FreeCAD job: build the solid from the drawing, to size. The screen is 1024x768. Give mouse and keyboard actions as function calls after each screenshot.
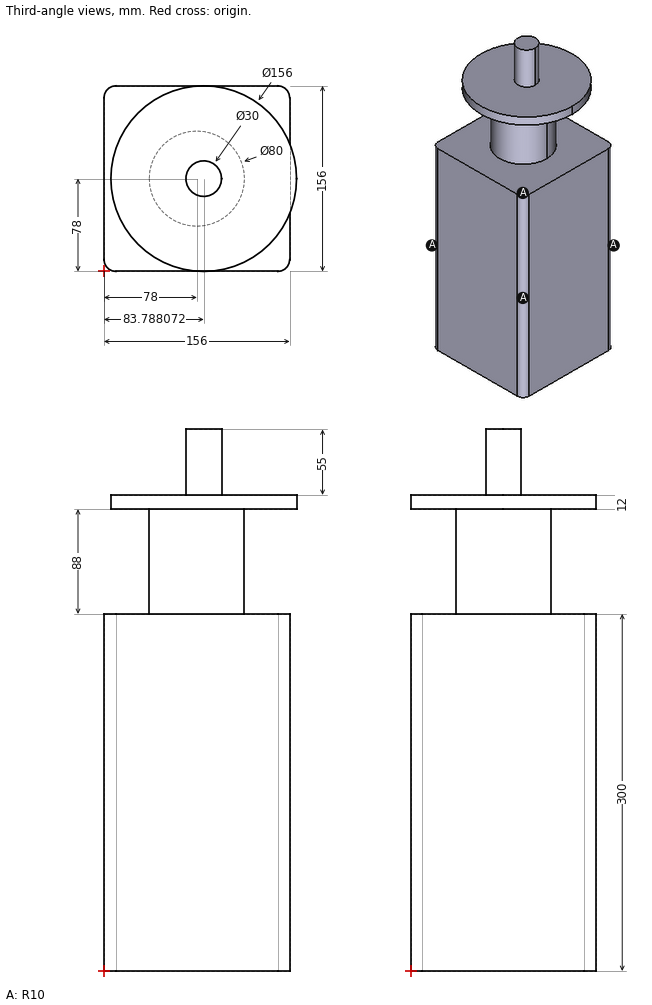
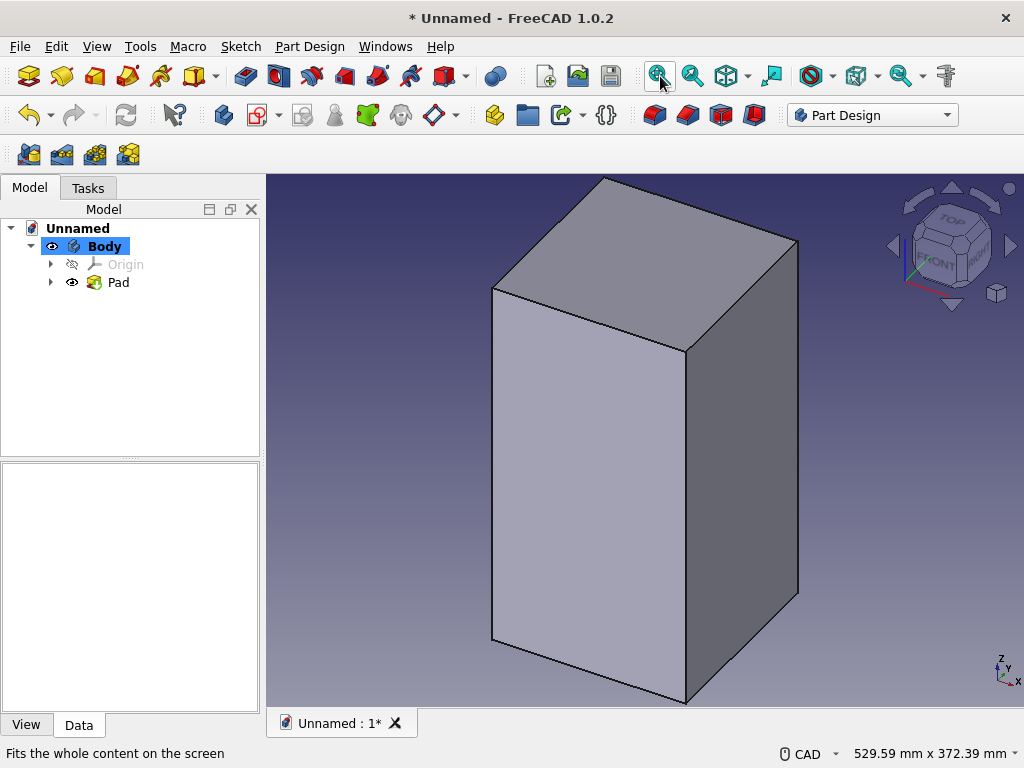
click(645, 264)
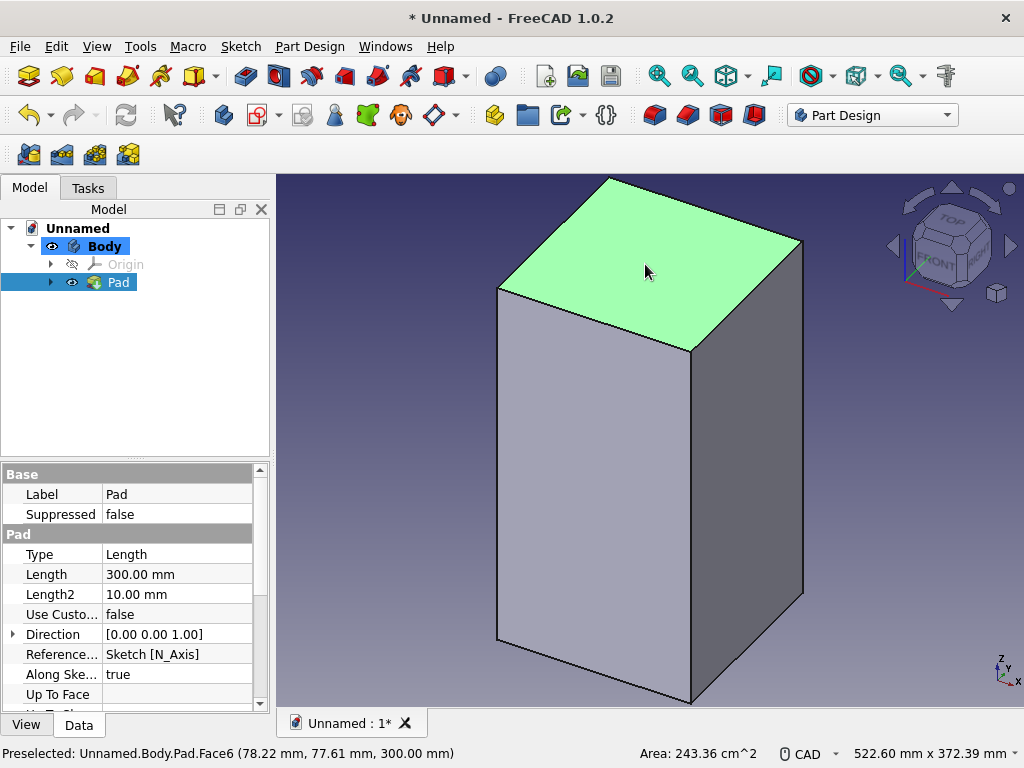
click(256, 116)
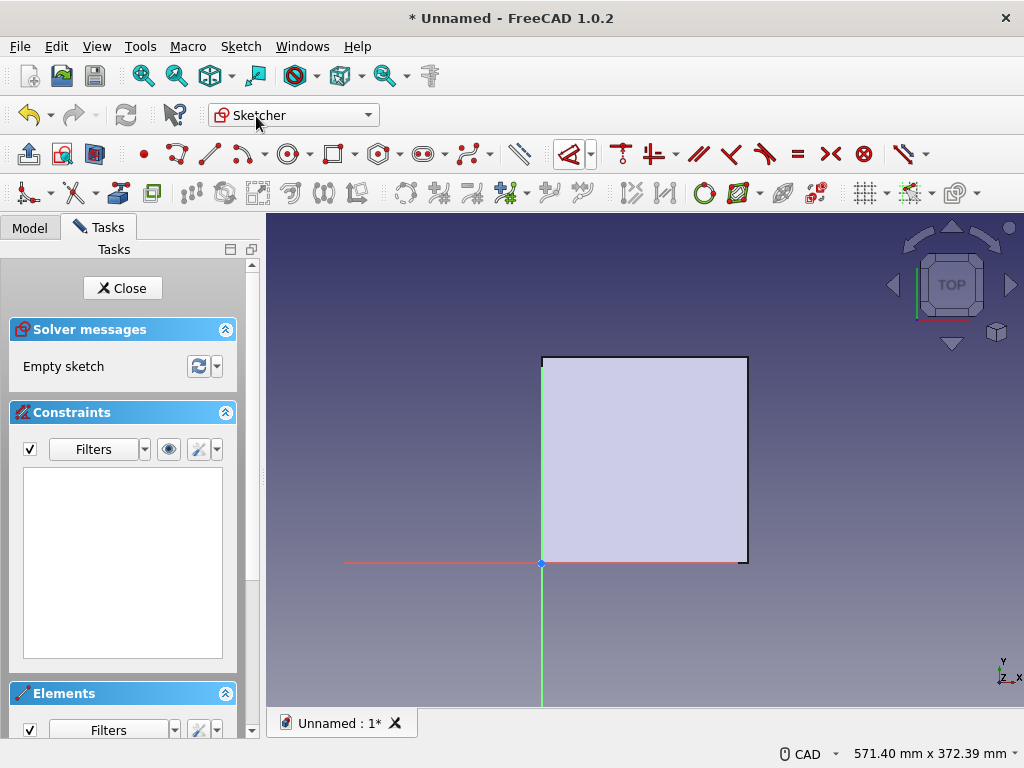
scroll(672, 516, up, 3)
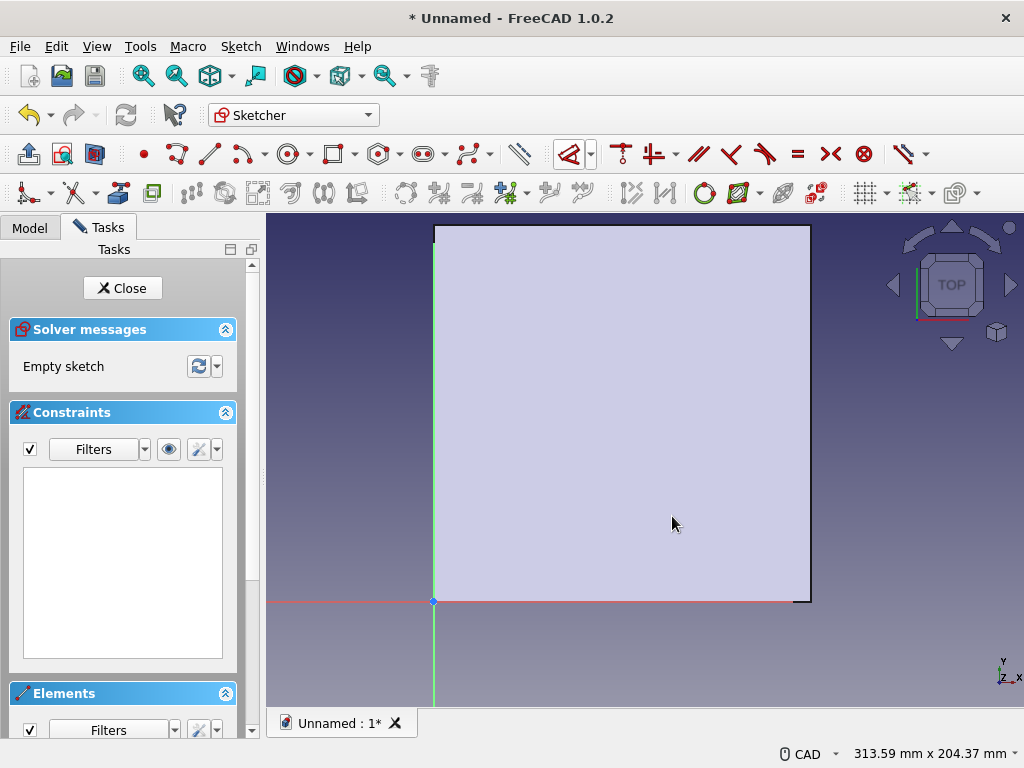
click(288, 154)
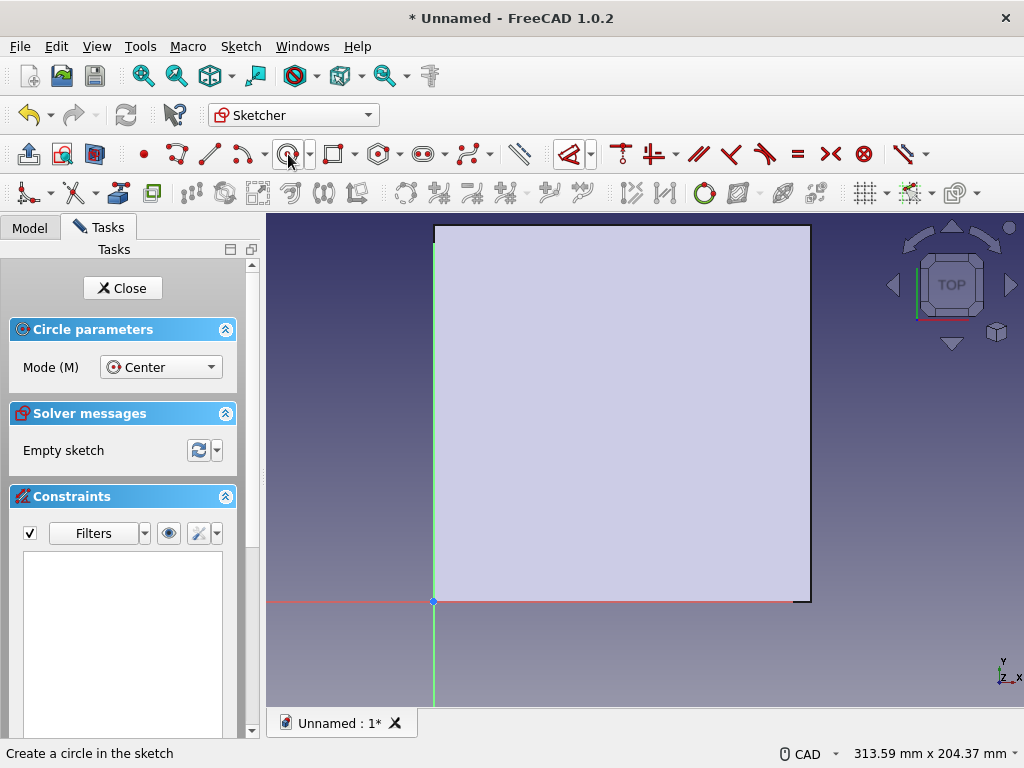
click(622, 413)
move(691, 345)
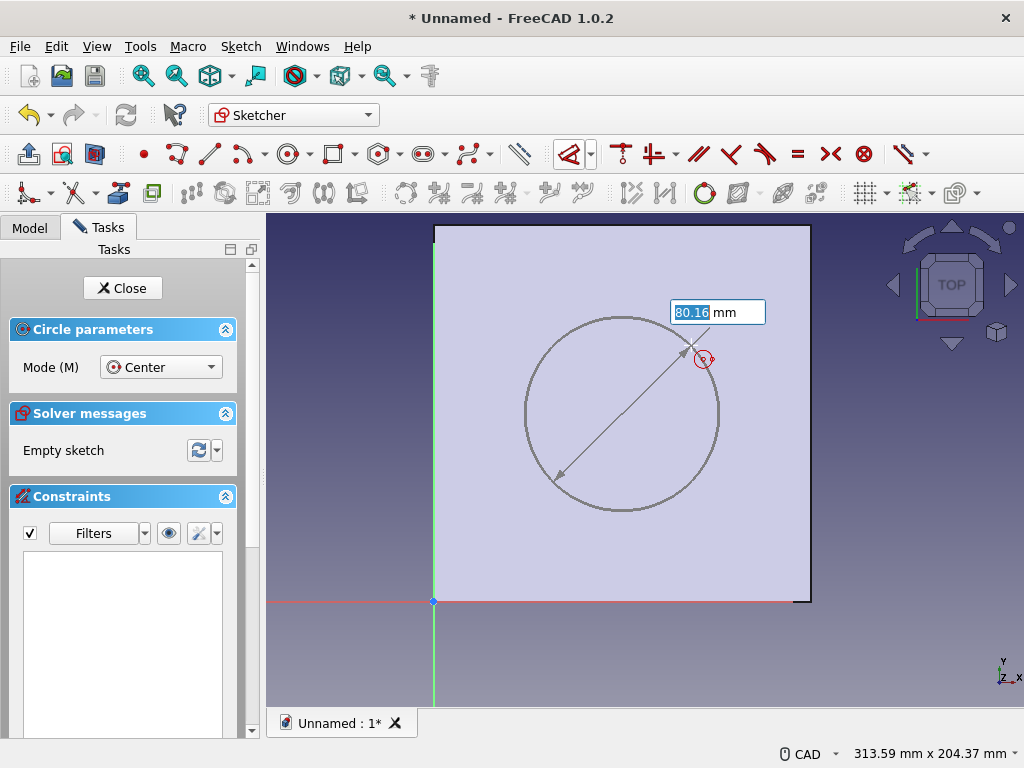
text(80)
key(Return)
key(Escape)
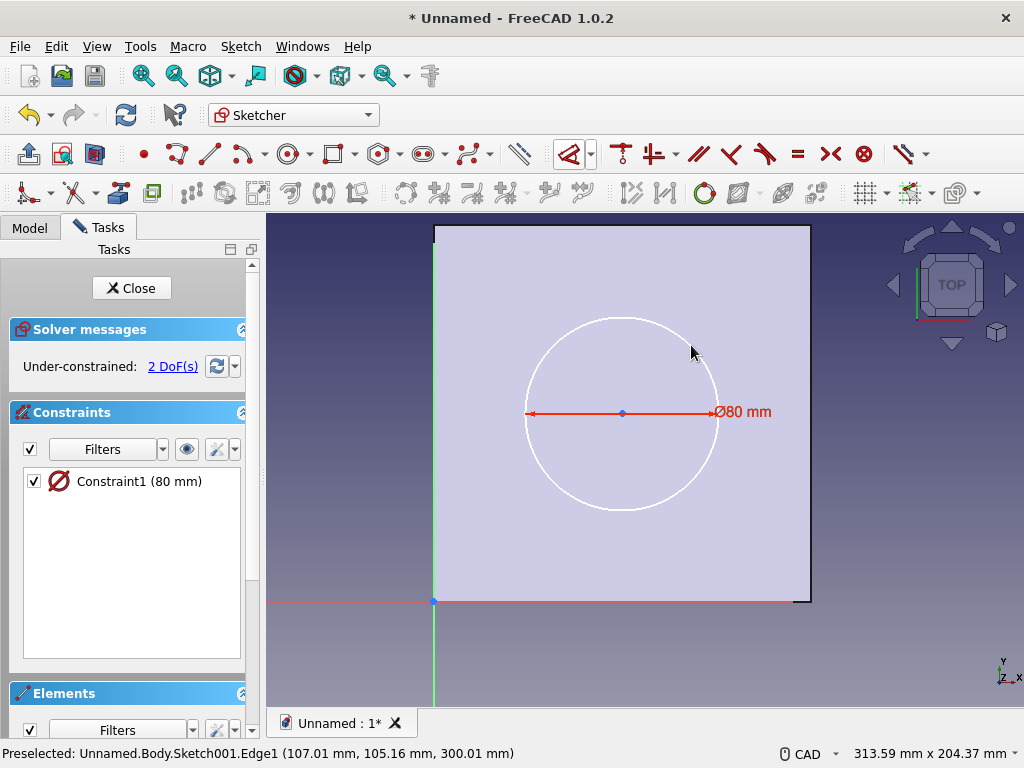
click(568, 154)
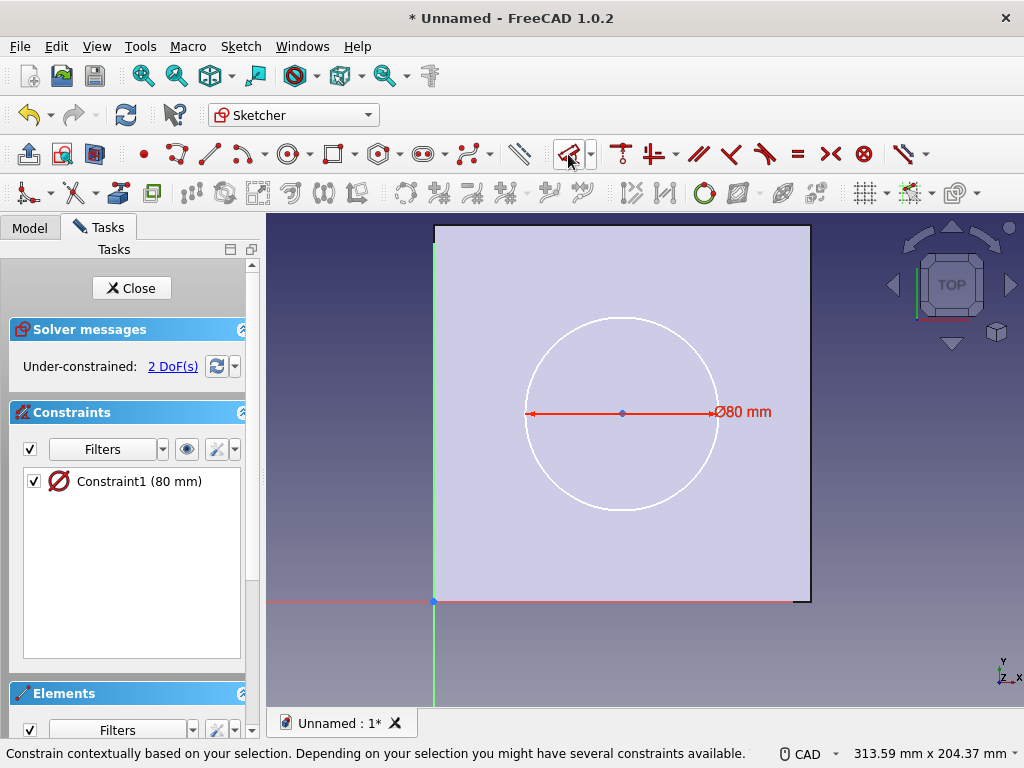
click(622, 414)
click(528, 636)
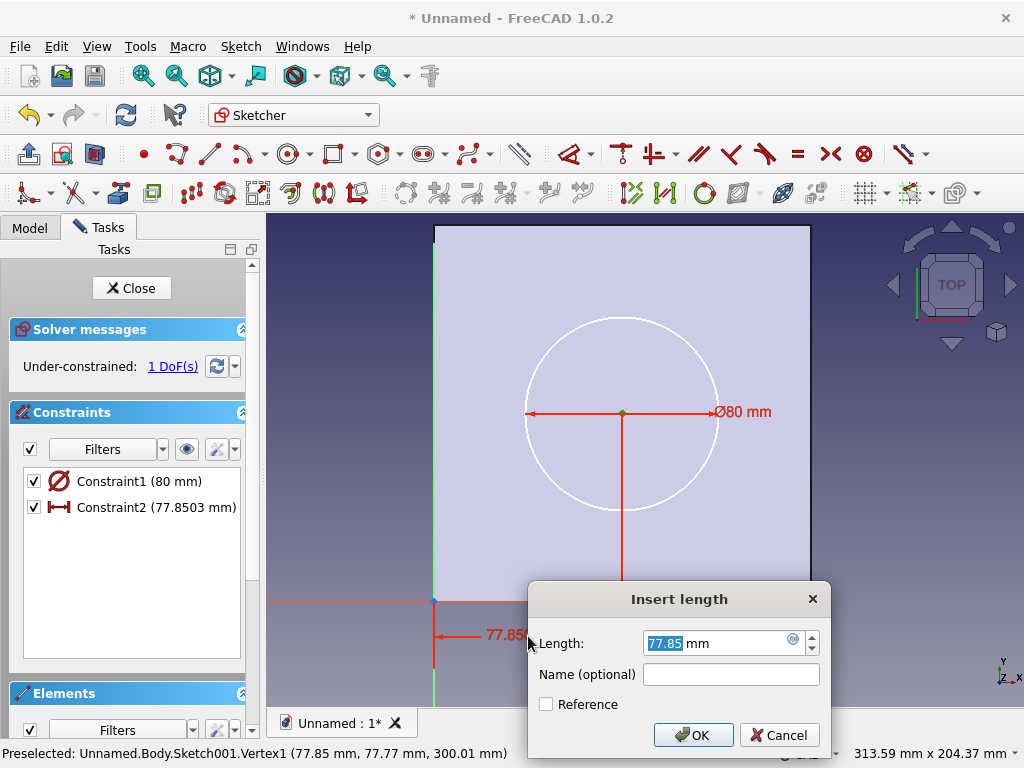
text(78)
key(Return)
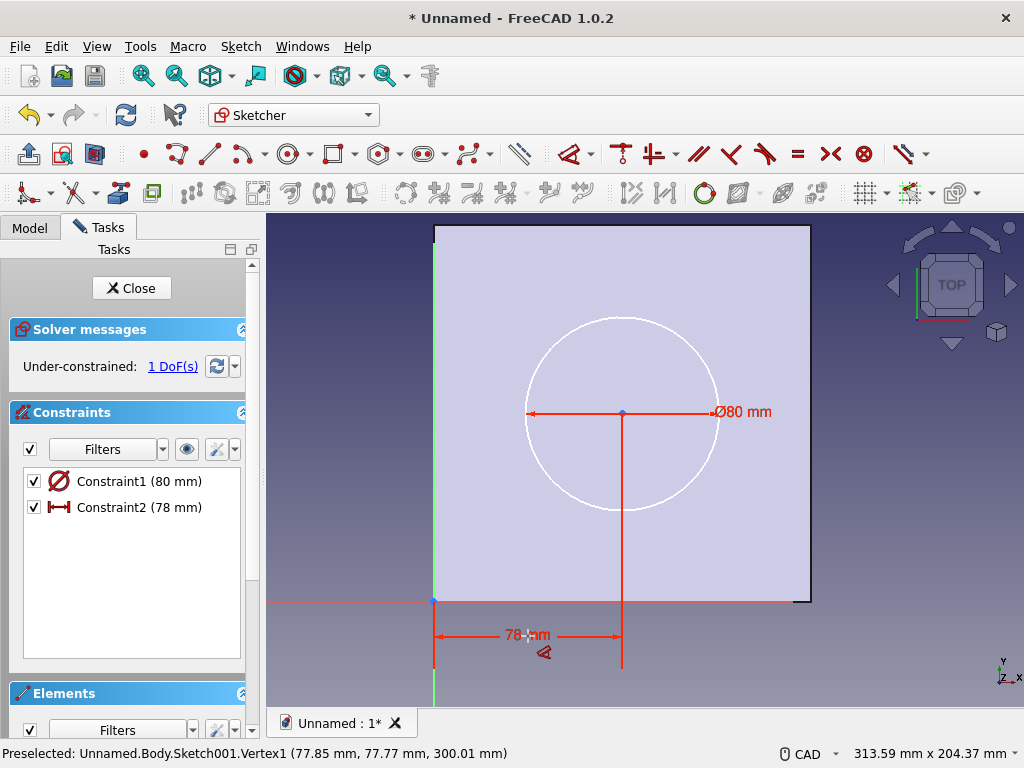
click(622, 414)
click(400, 508)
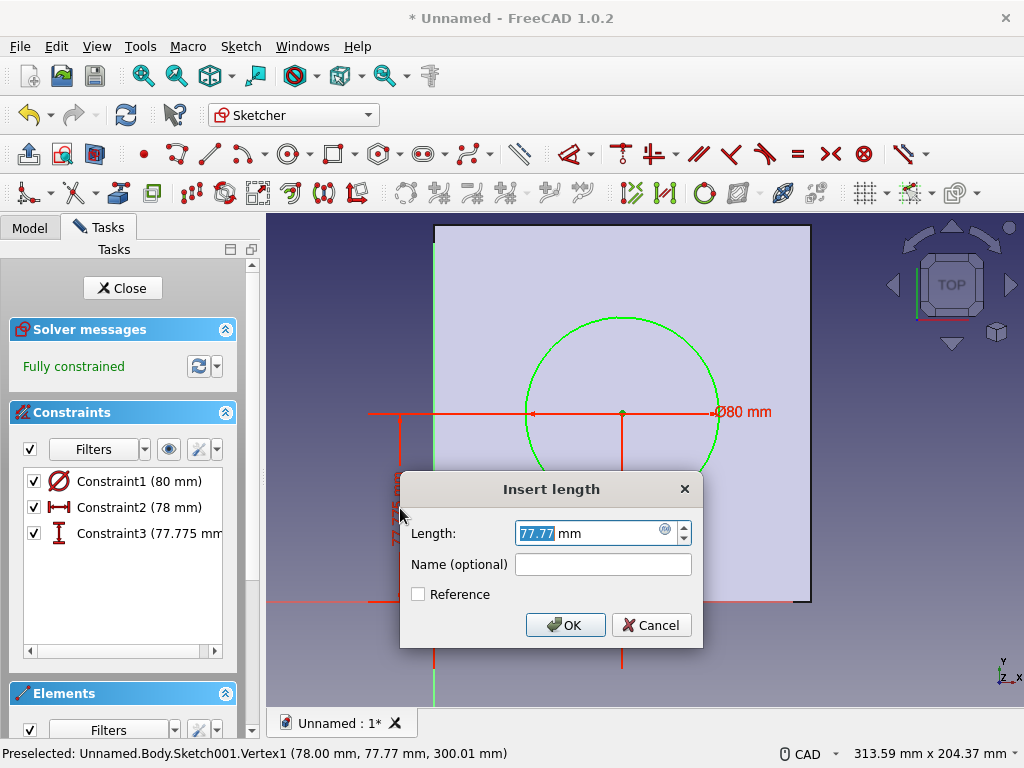
text(78)
key(Return)
key(Escape)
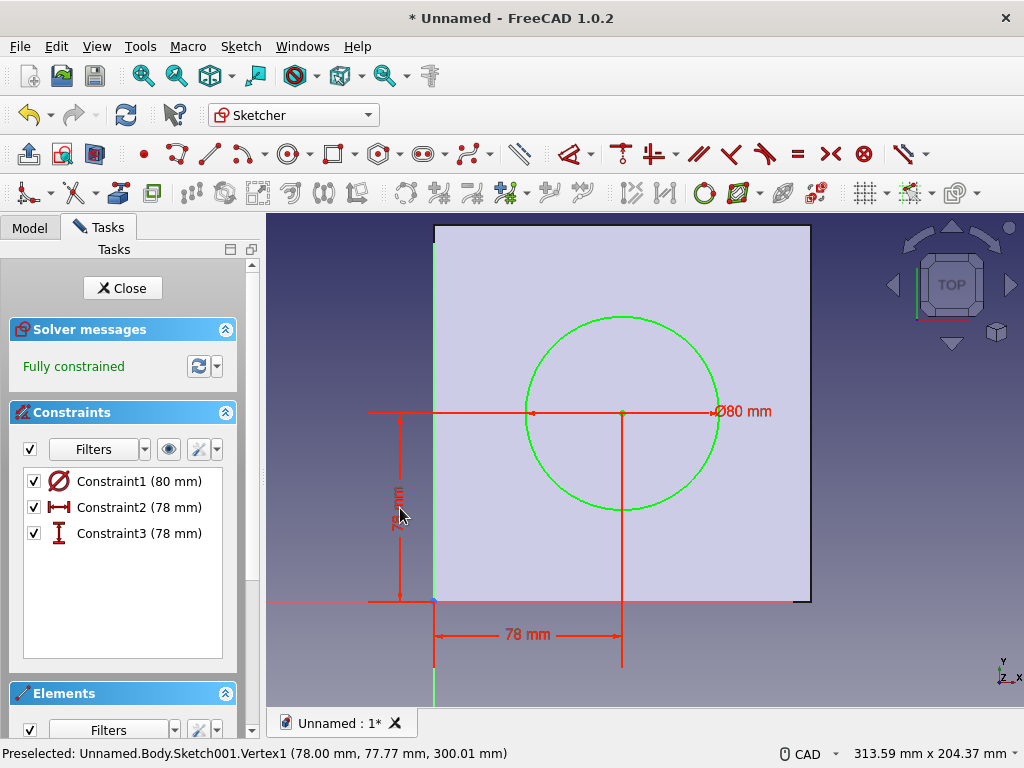
click(123, 288)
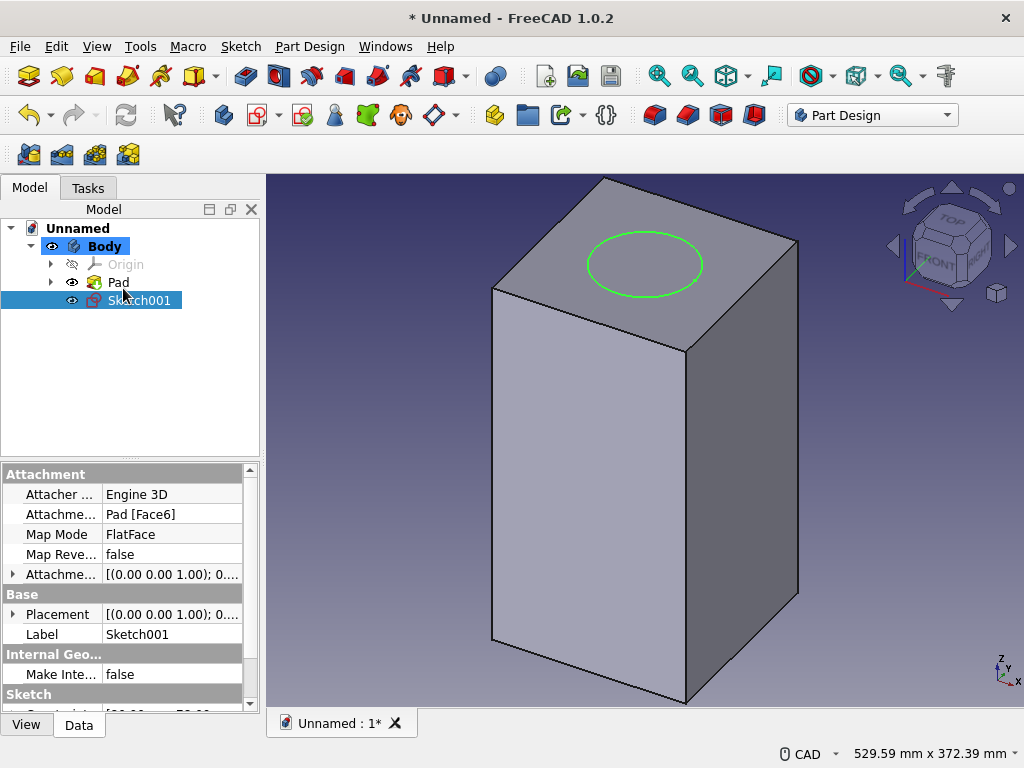
click(29, 76)